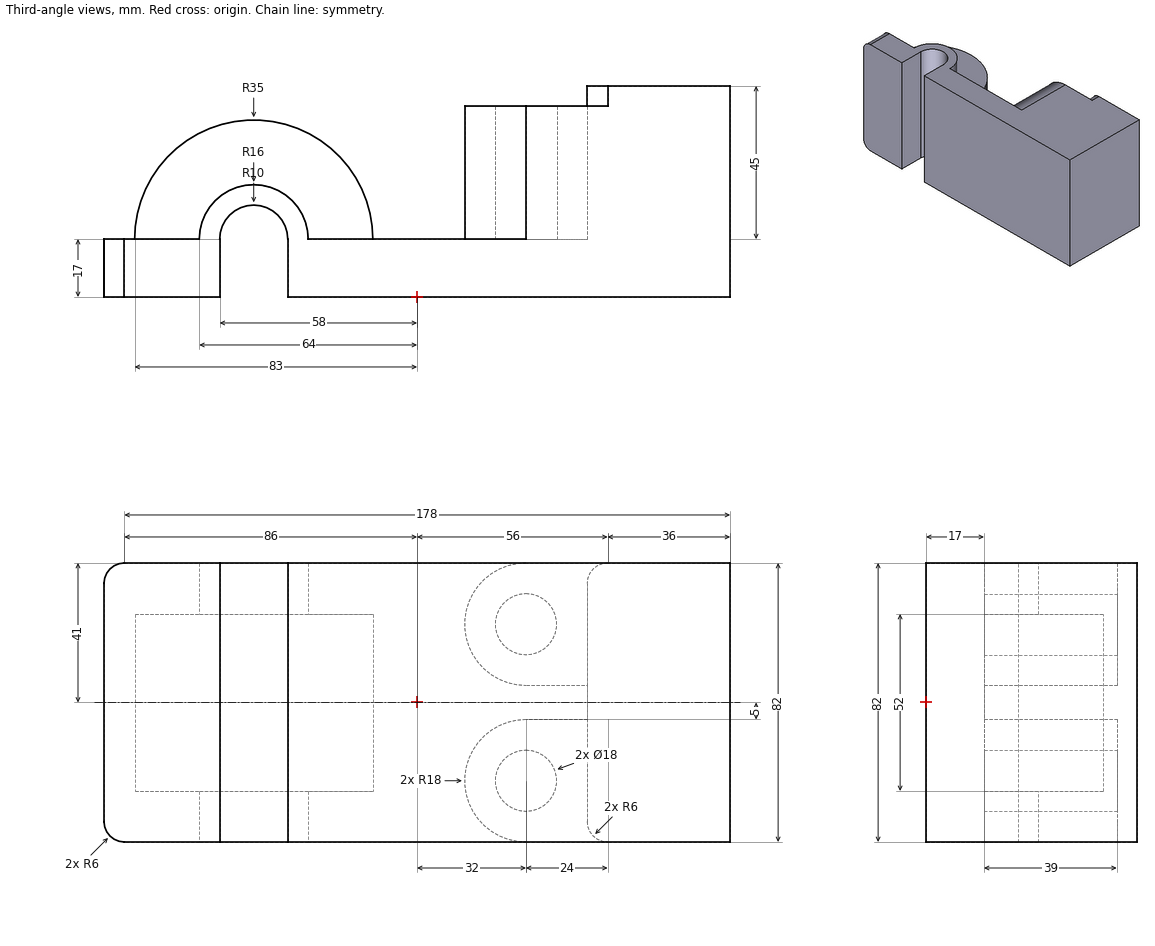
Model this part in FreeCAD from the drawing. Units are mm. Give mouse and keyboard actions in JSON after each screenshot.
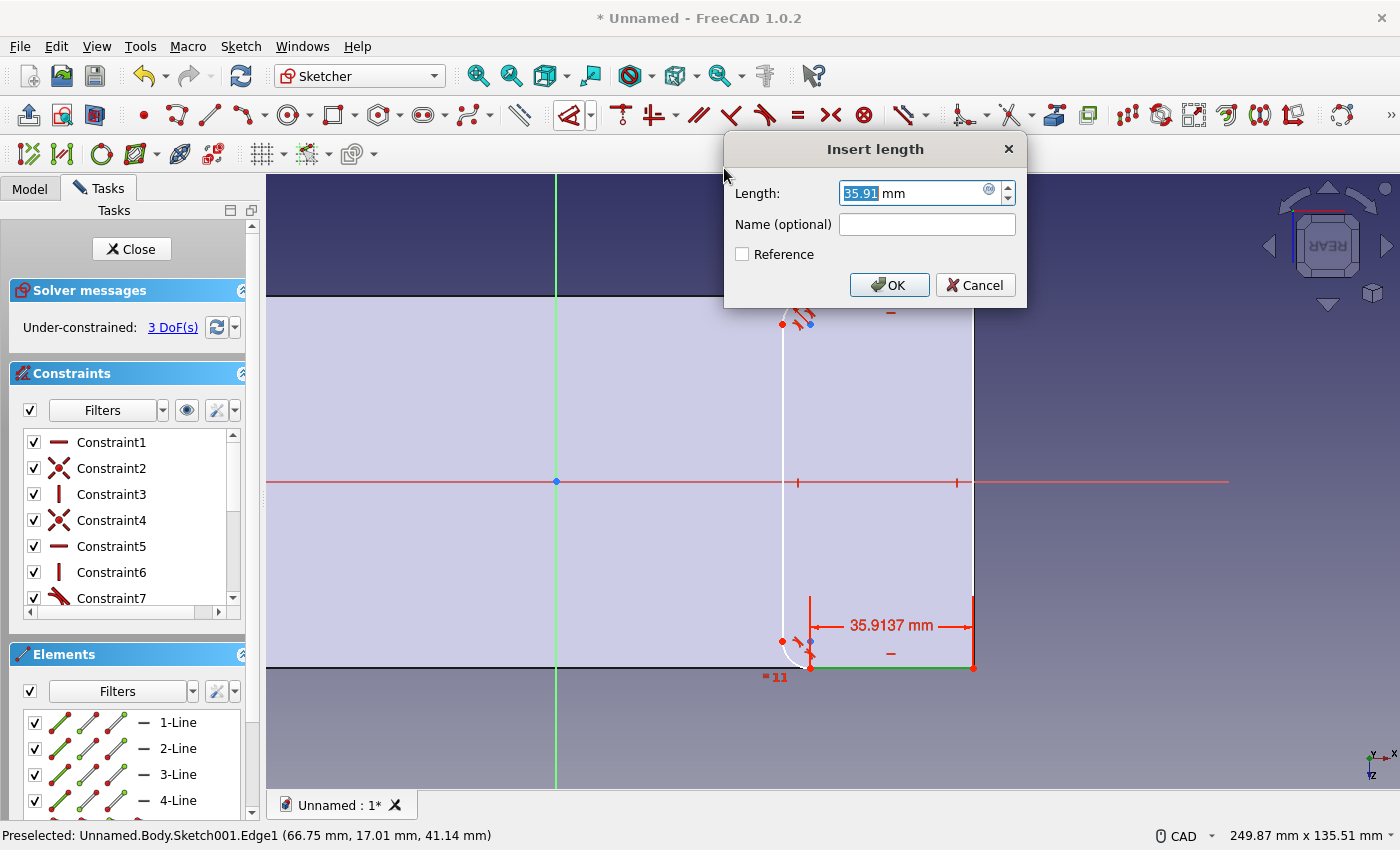
{"action": "type", "text": "36"}
{"action": "key", "text": "Return"}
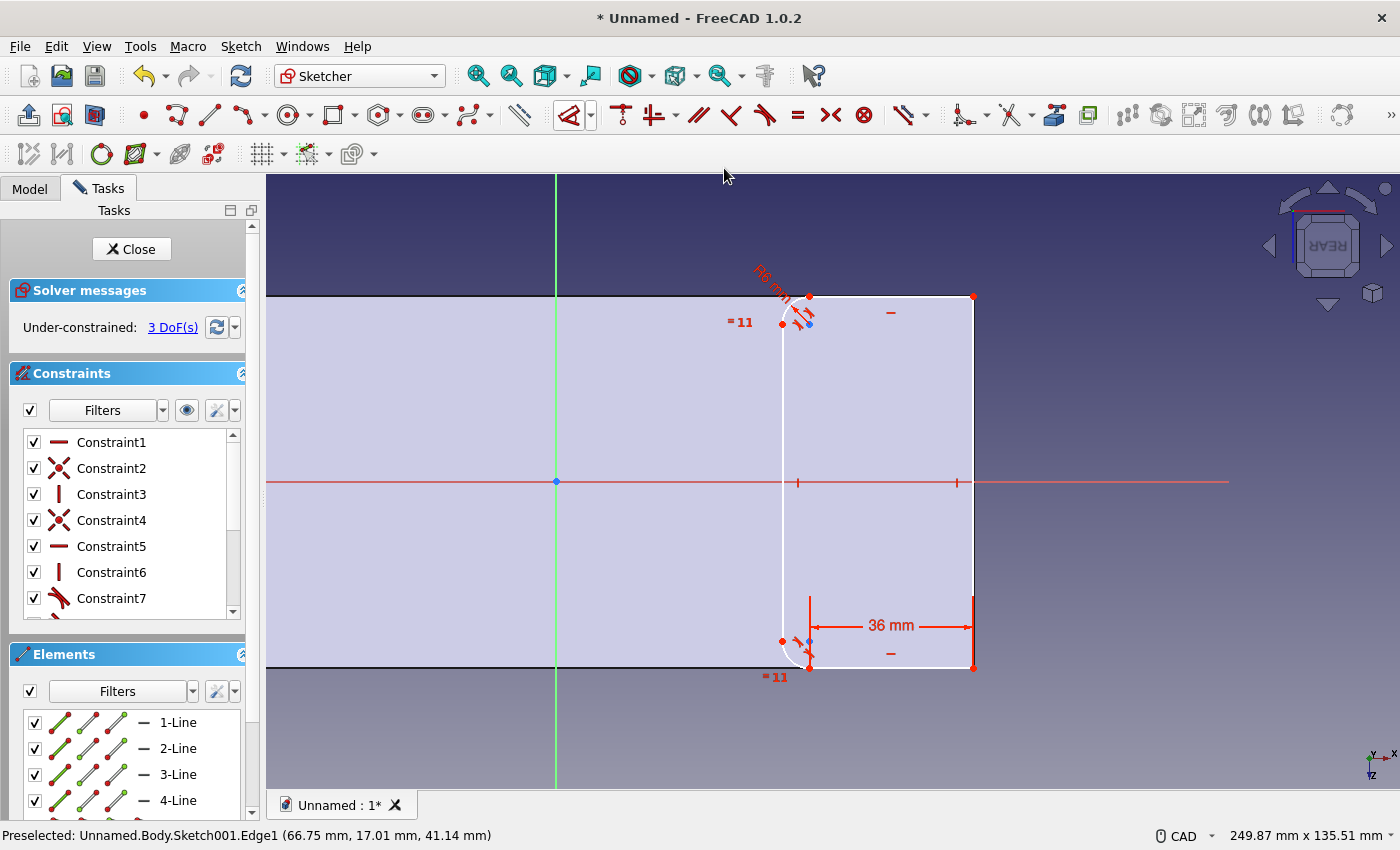
{"action": "left_click", "coordinate": [973, 557]}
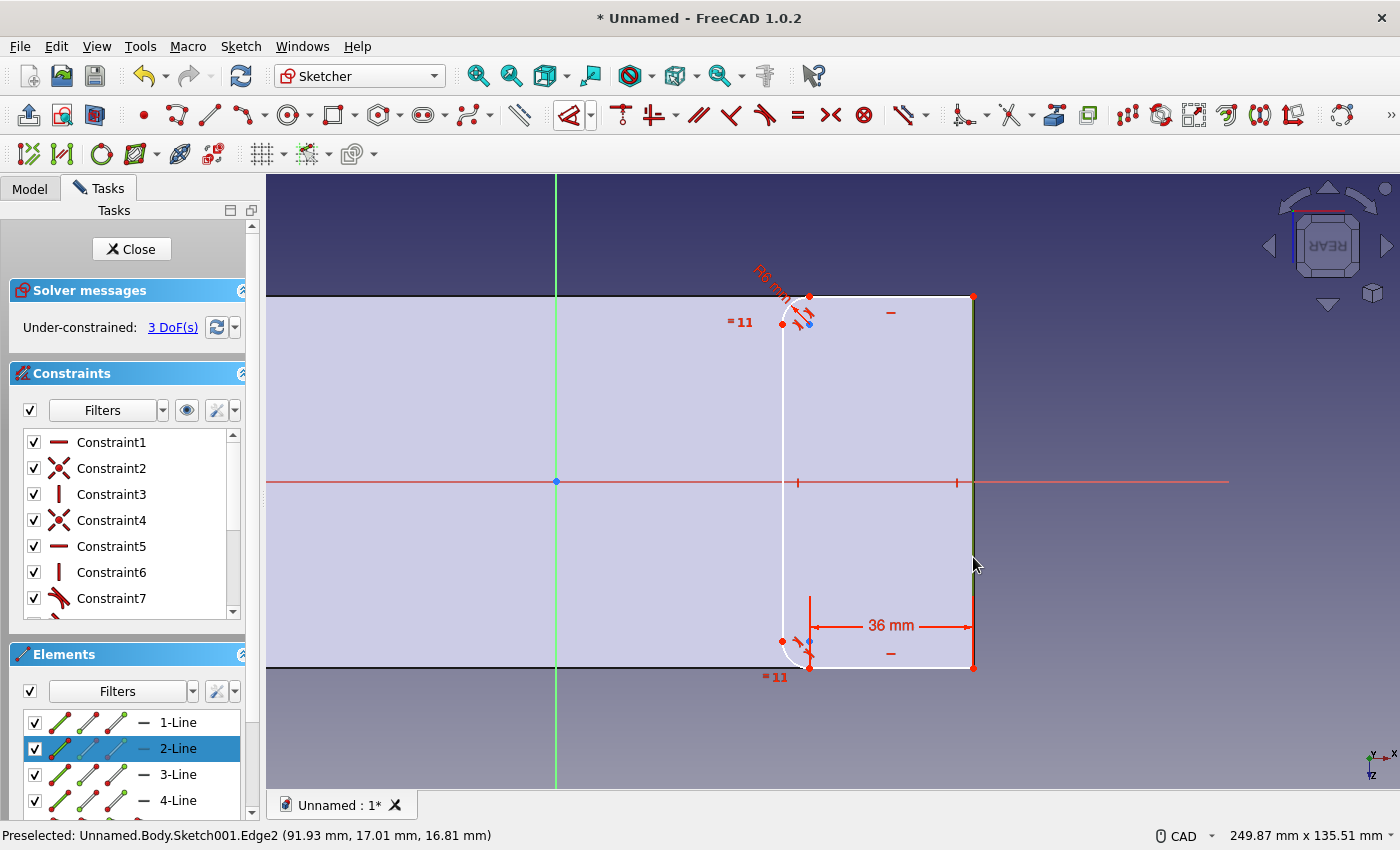
{"action": "key", "text": "i"}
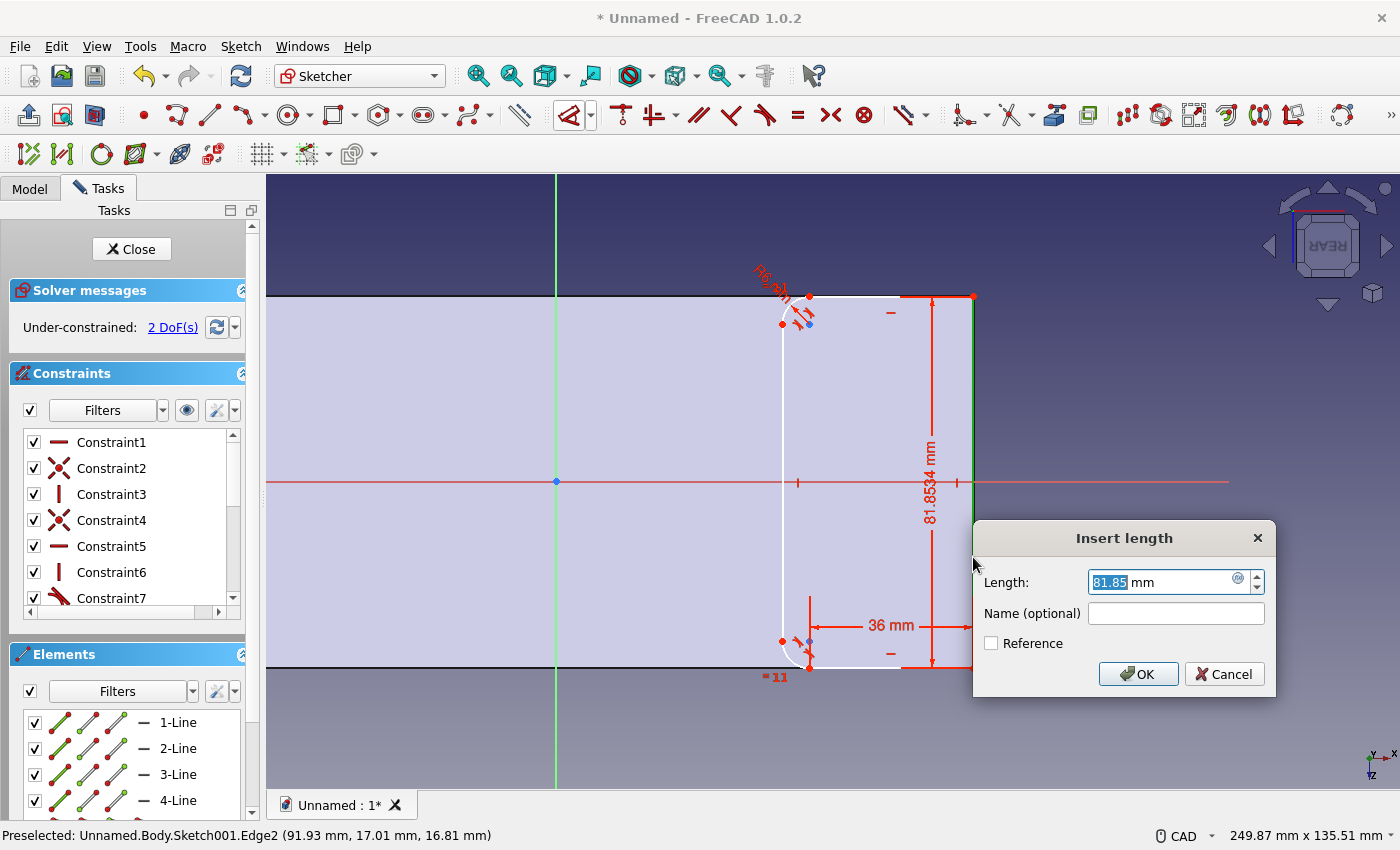
{"action": "type", "text": "82"}
{"action": "key", "text": "Return"}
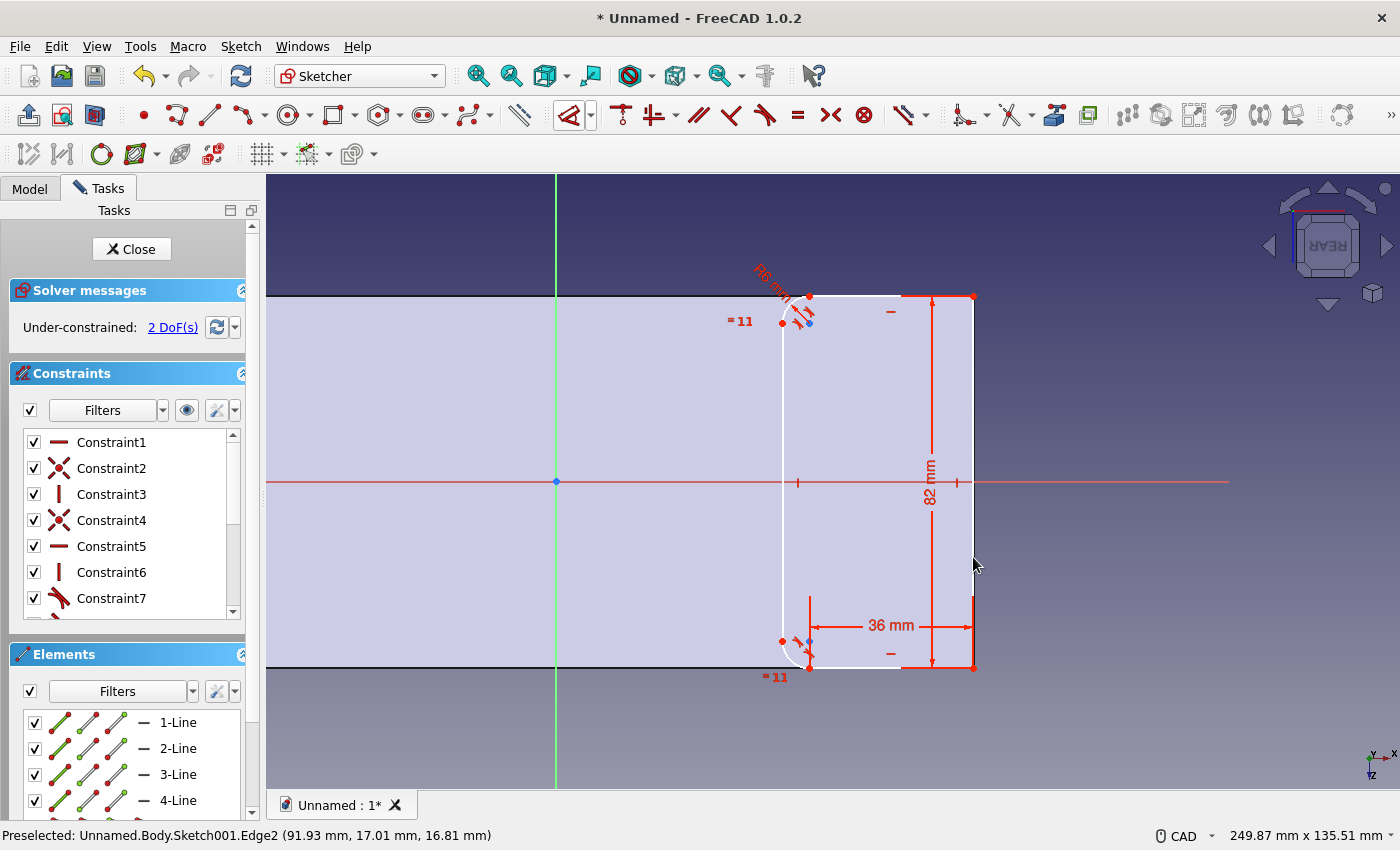
{"action": "left_click", "coordinate": [810, 668]}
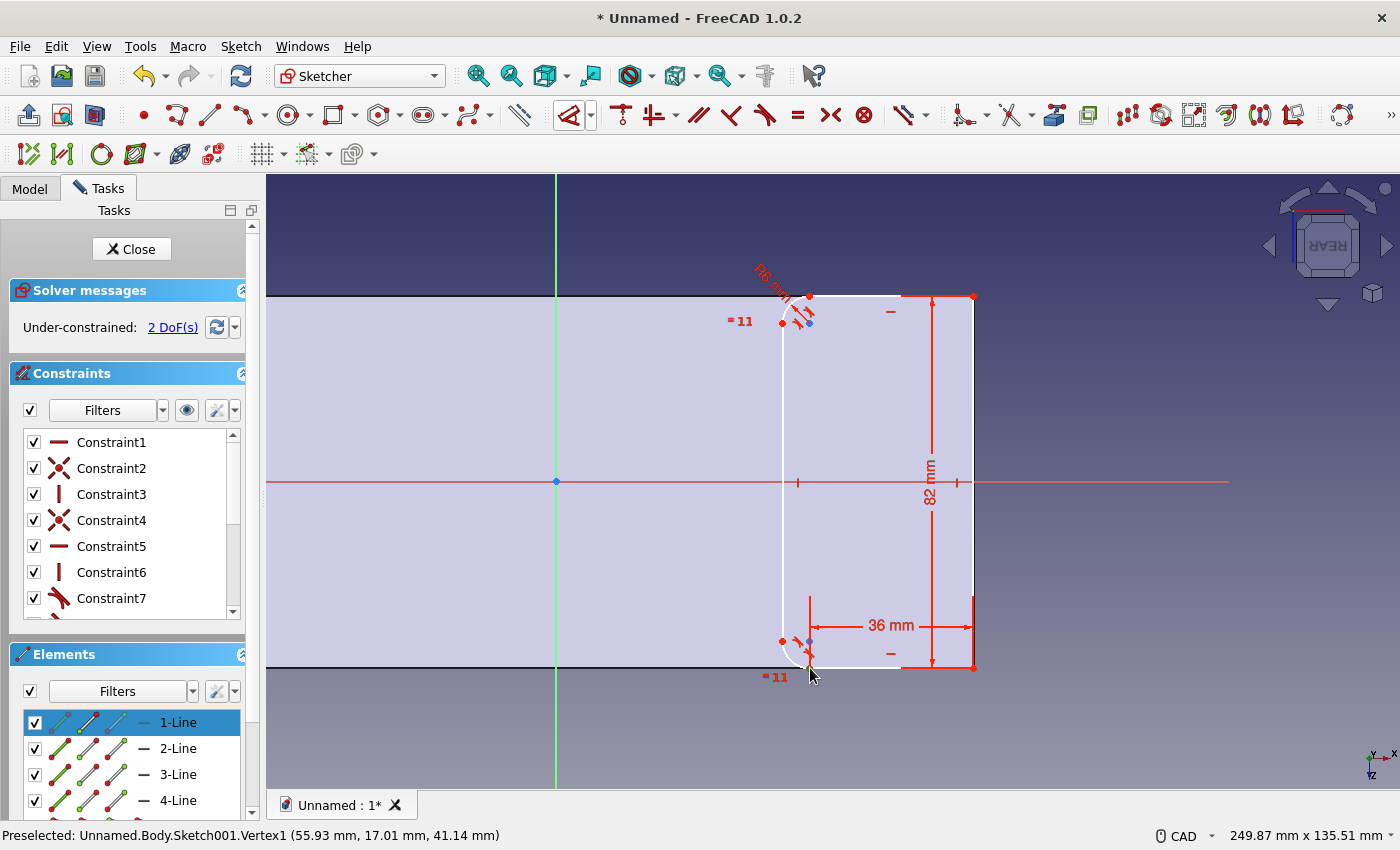
{"action": "left_click", "coordinate": [590, 116]}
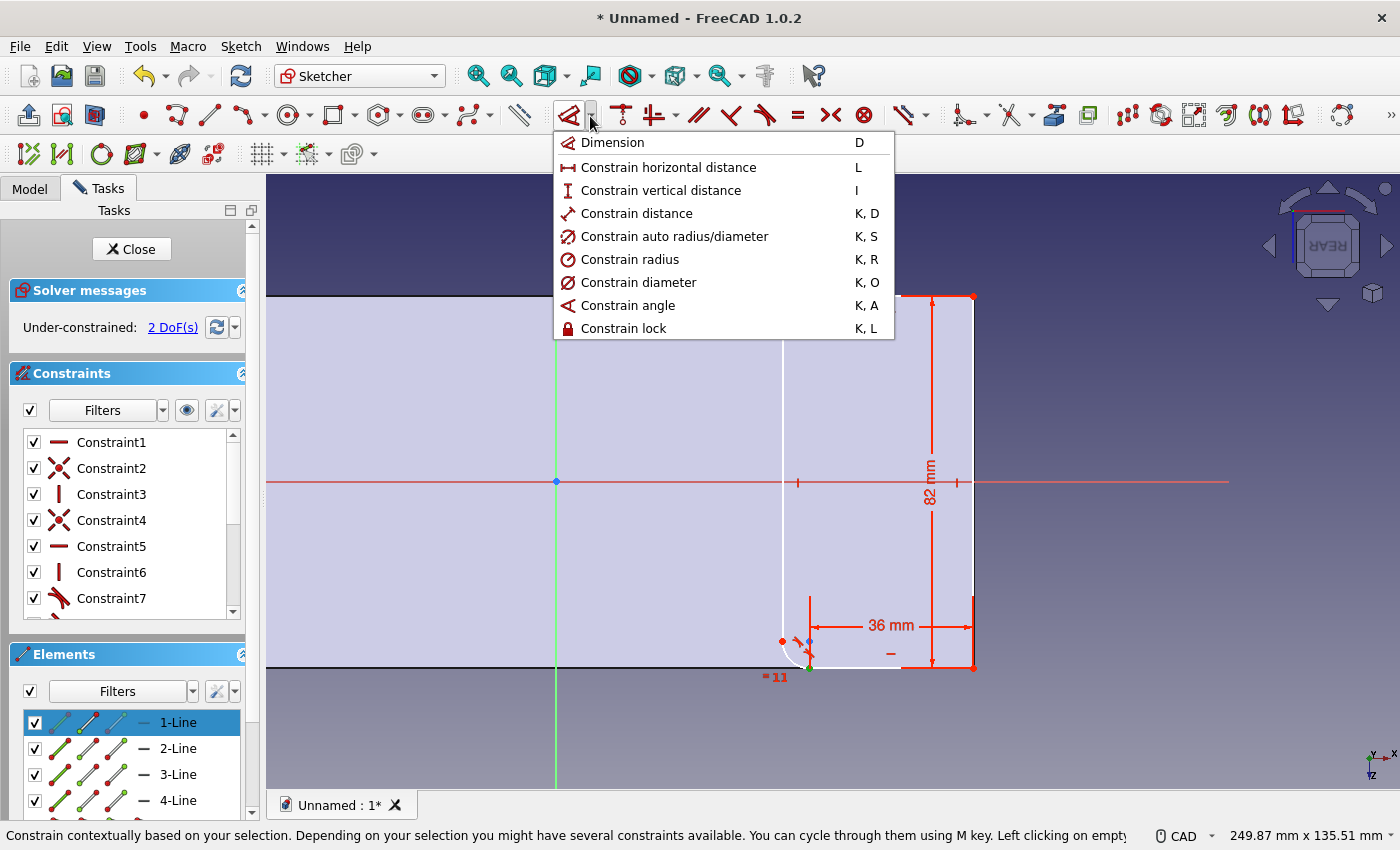
{"action": "left_click", "coordinate": [724, 168]}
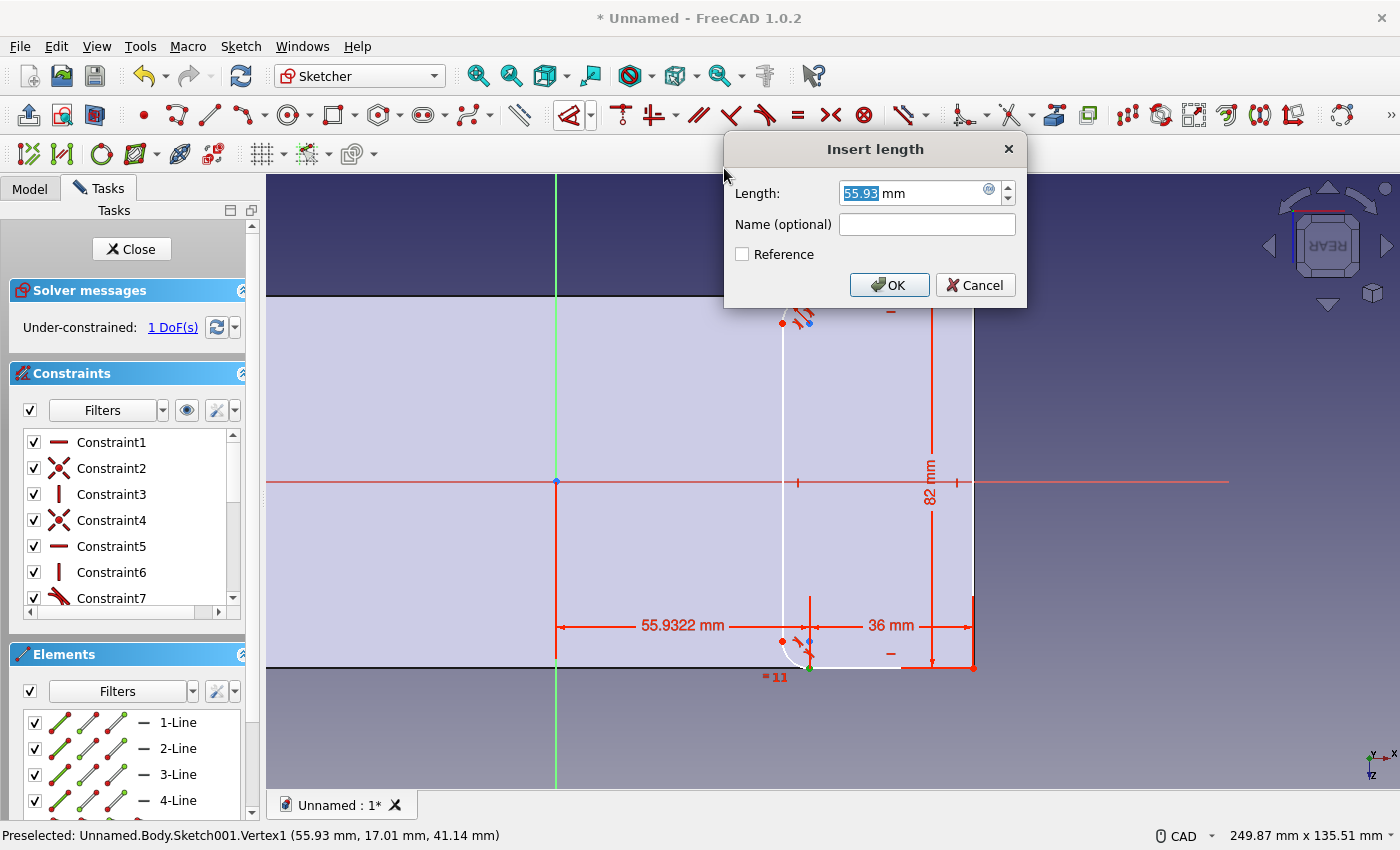
{"action": "type", "text": "56"}
{"action": "key", "text": "Return"}